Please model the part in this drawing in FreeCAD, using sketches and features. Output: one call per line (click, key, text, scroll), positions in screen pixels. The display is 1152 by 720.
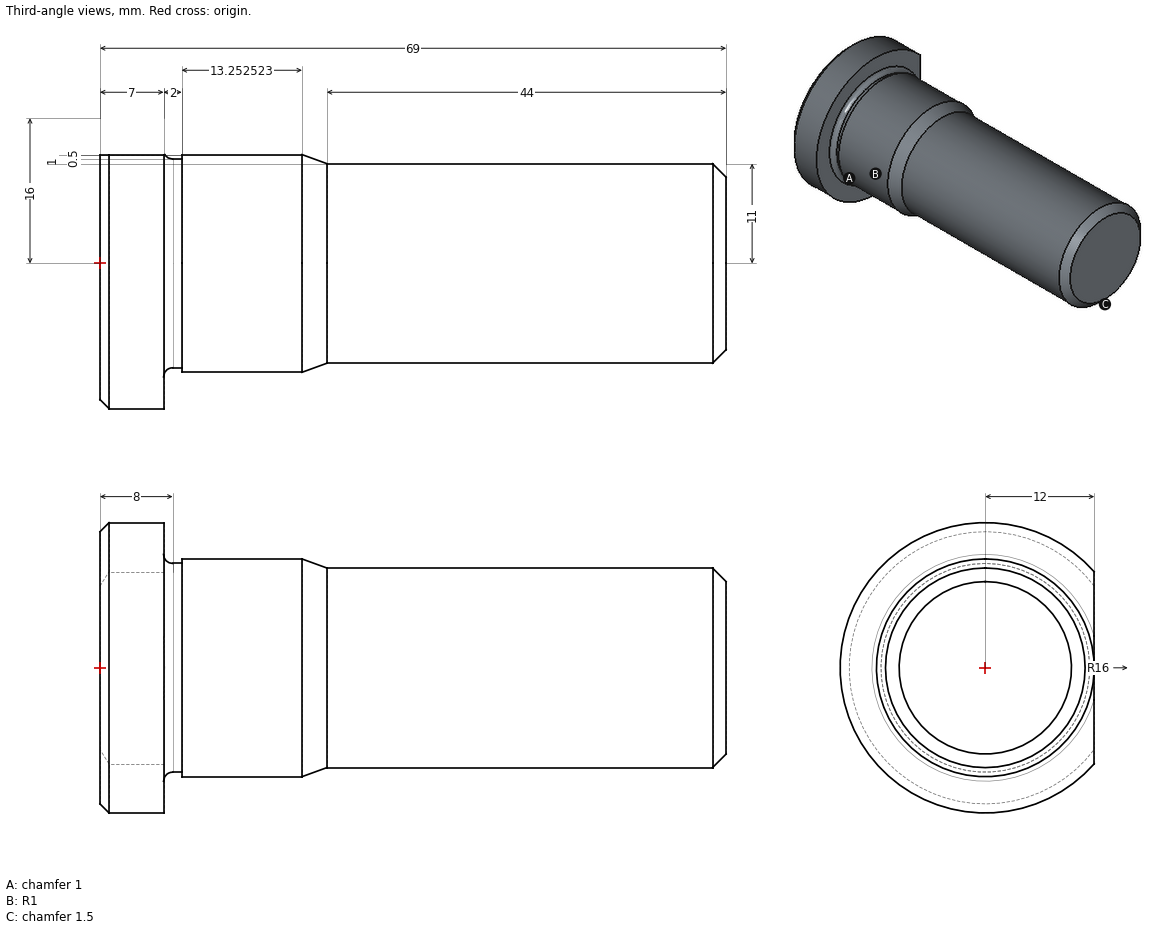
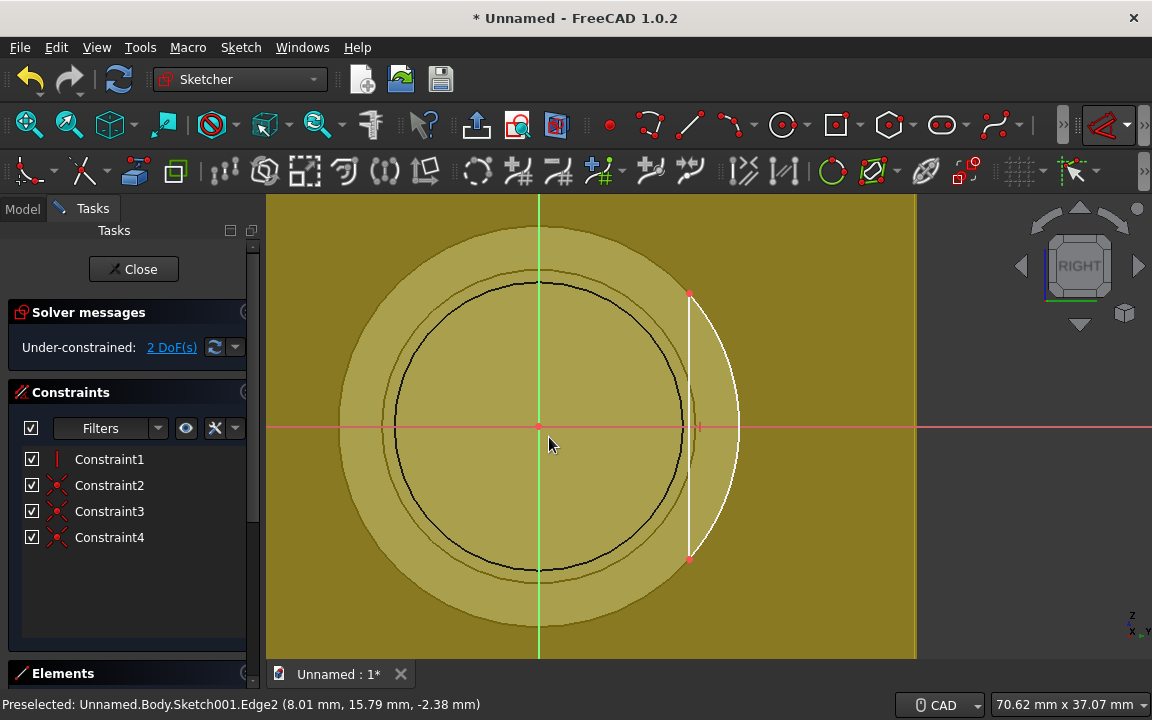
click(1102, 126)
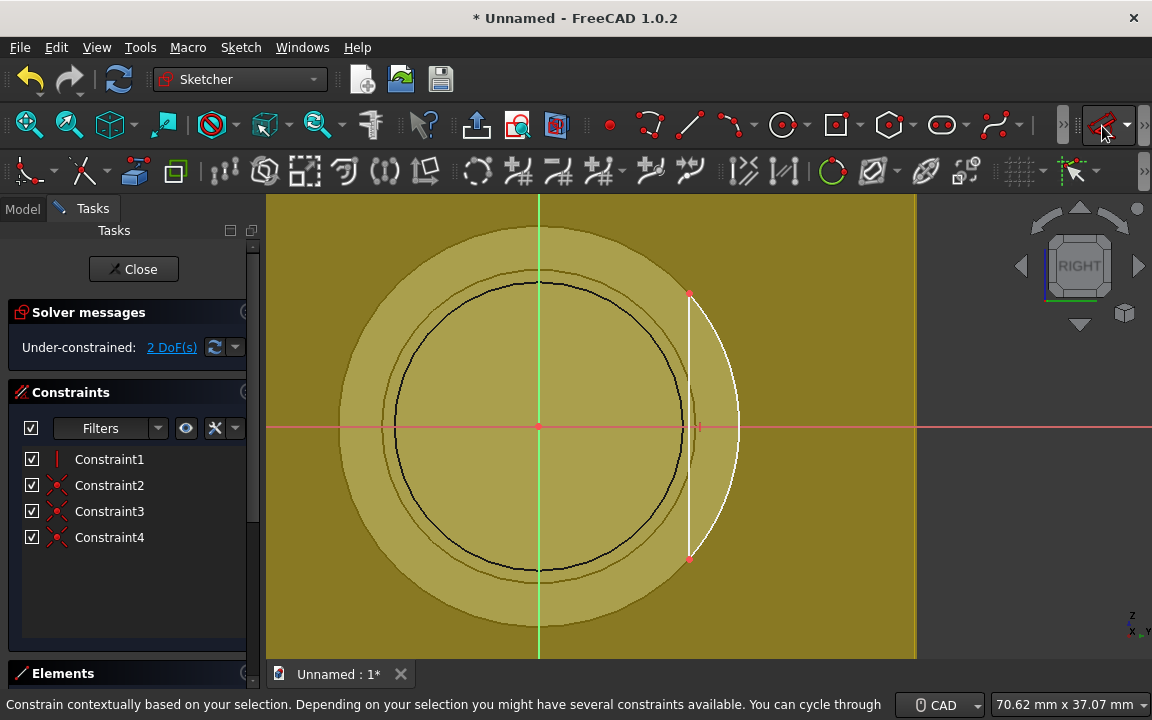
click(731, 484)
click(762, 493)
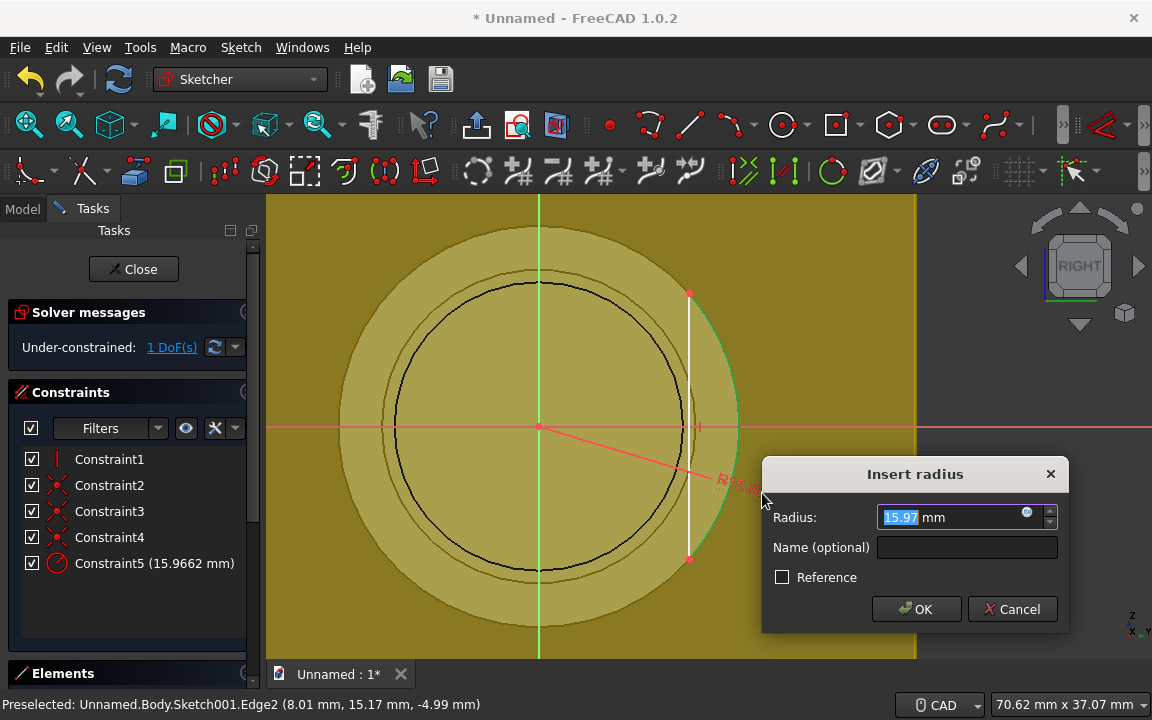
text(16)
key(Return)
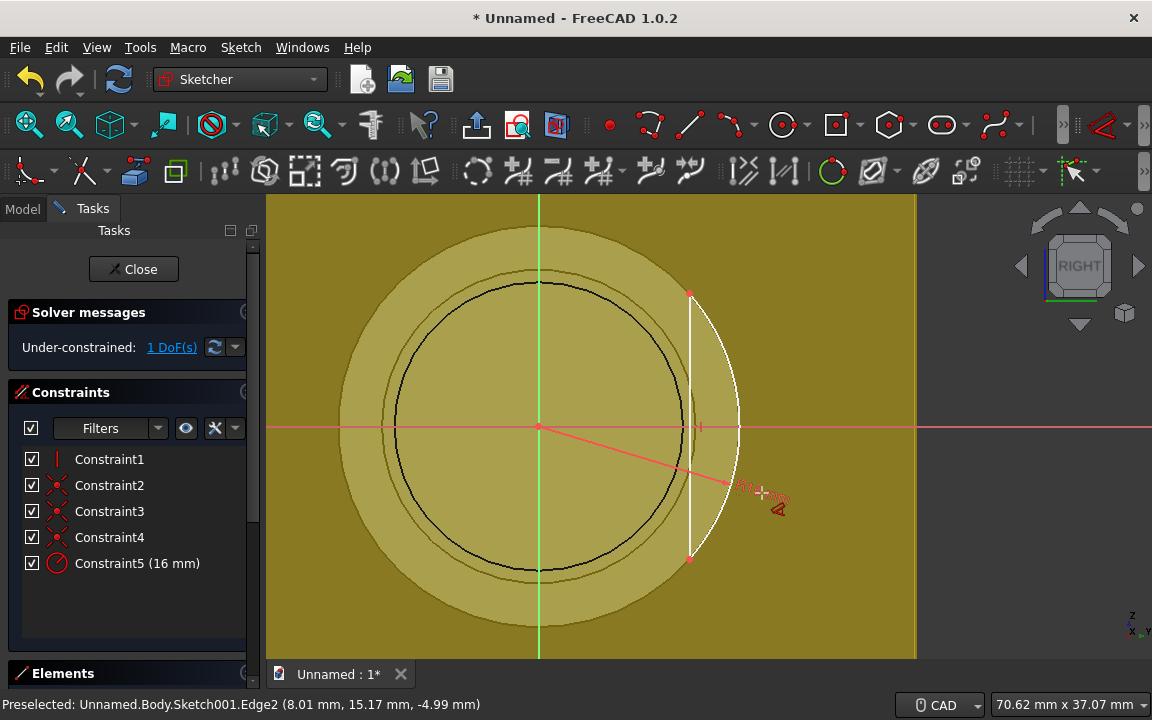
click(690, 294)
click(614, 260)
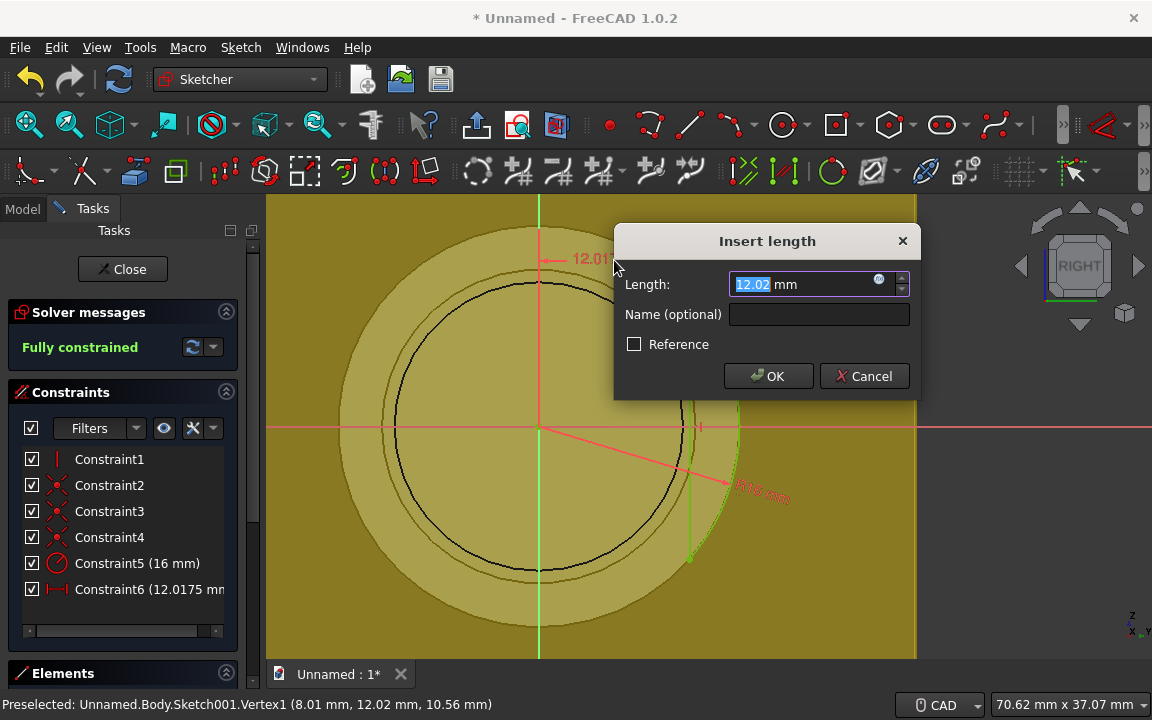
text(12)
key(Return)
key(Escape)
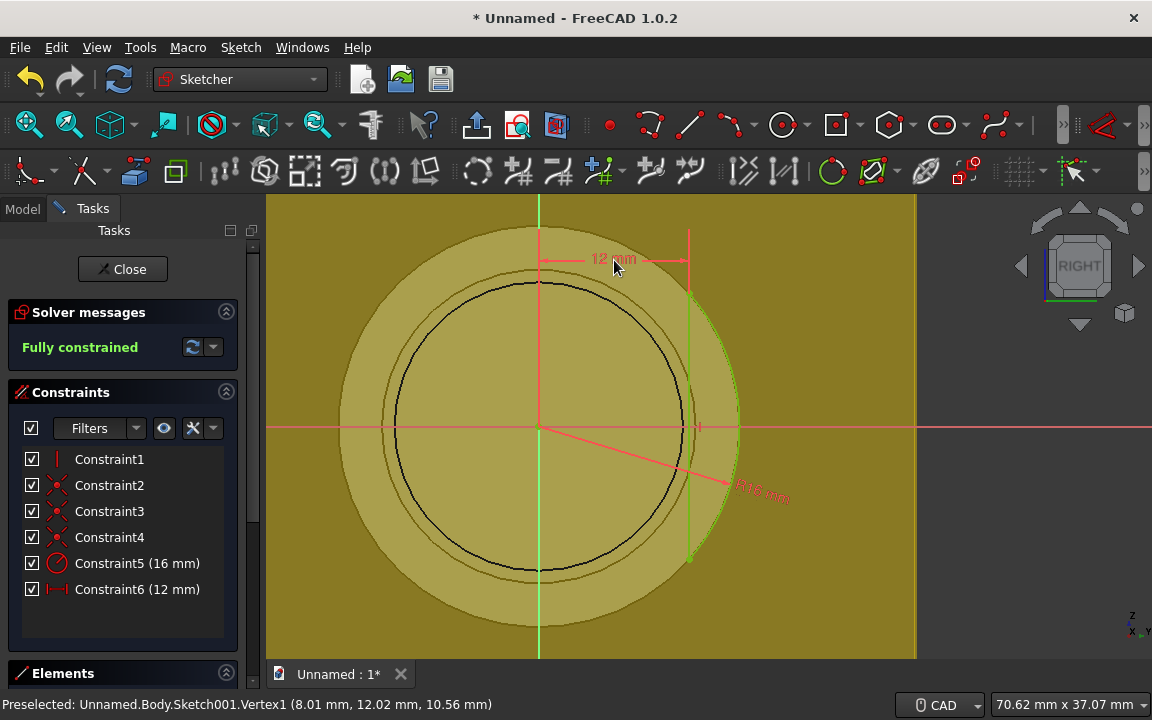
click(123, 269)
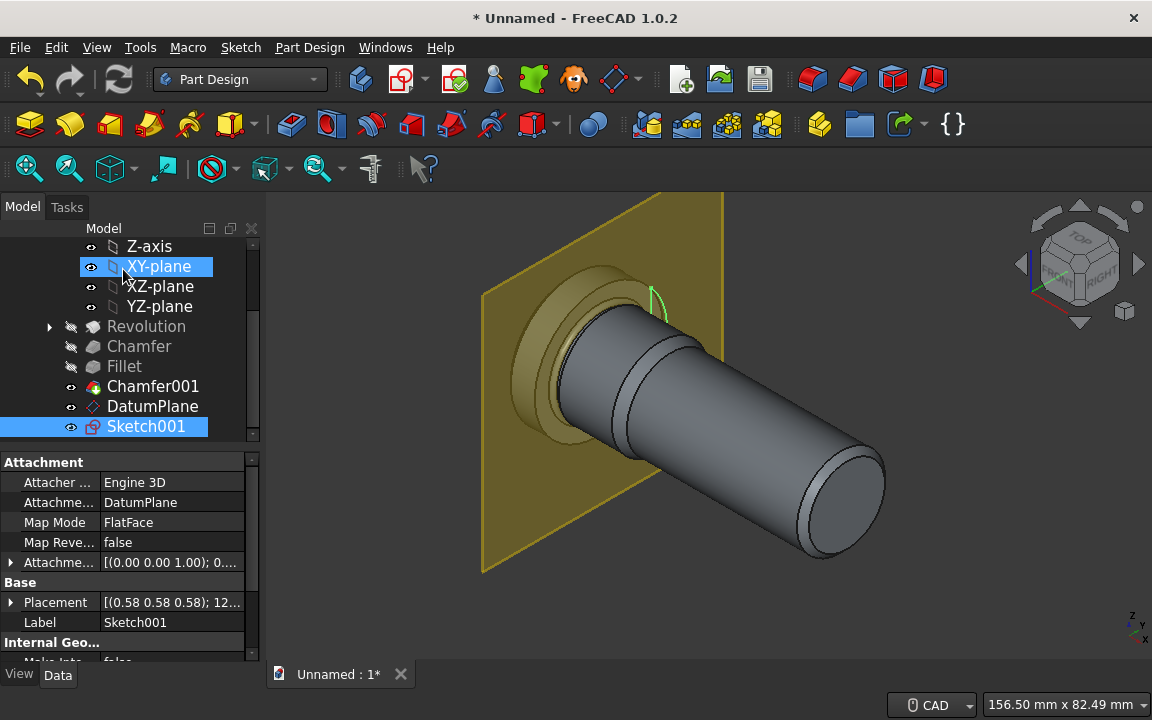
click(292, 124)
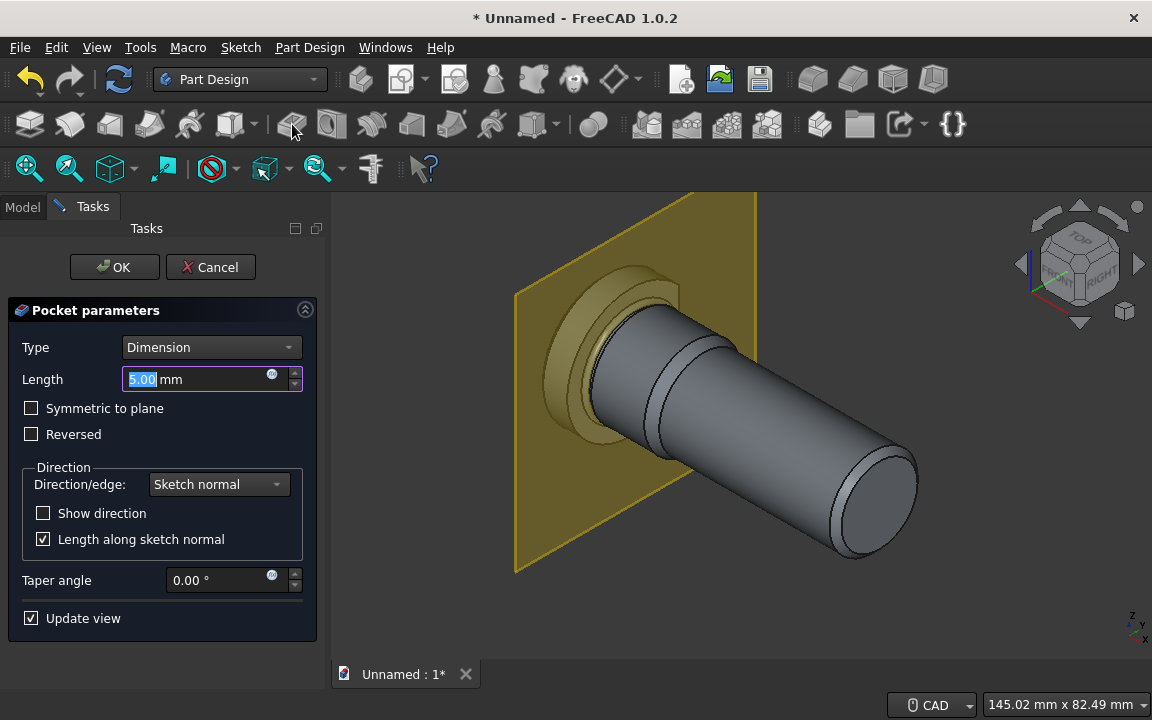
text(8)
key(Tab)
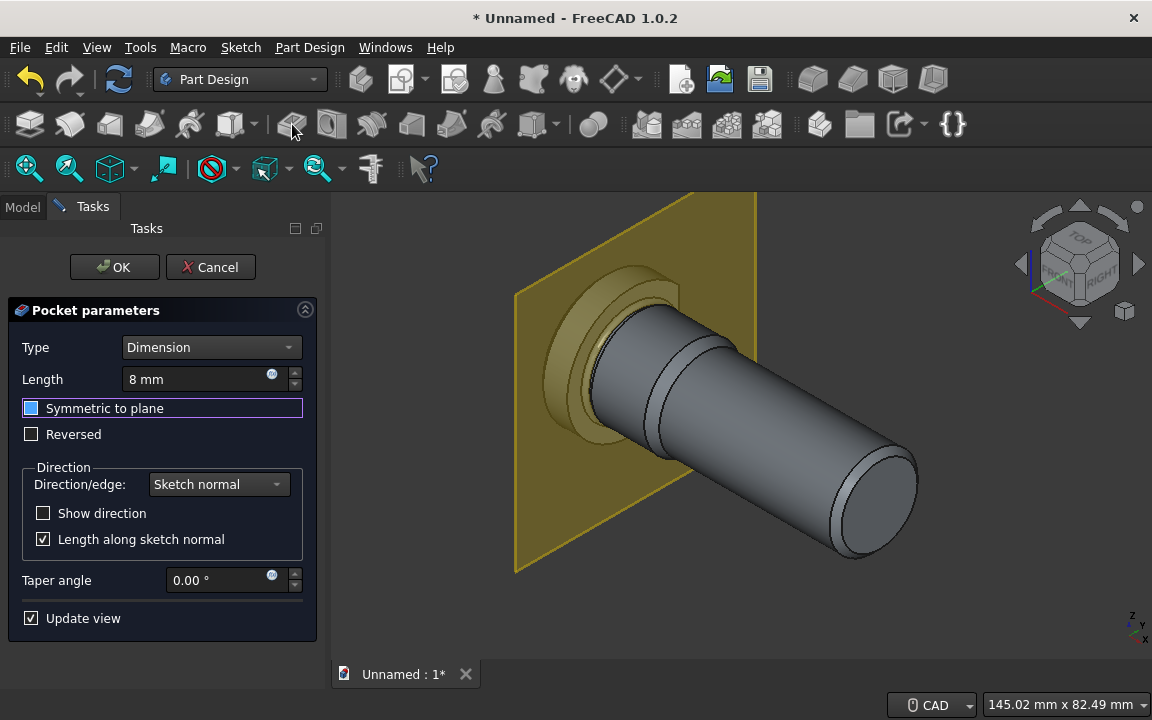
click(115, 267)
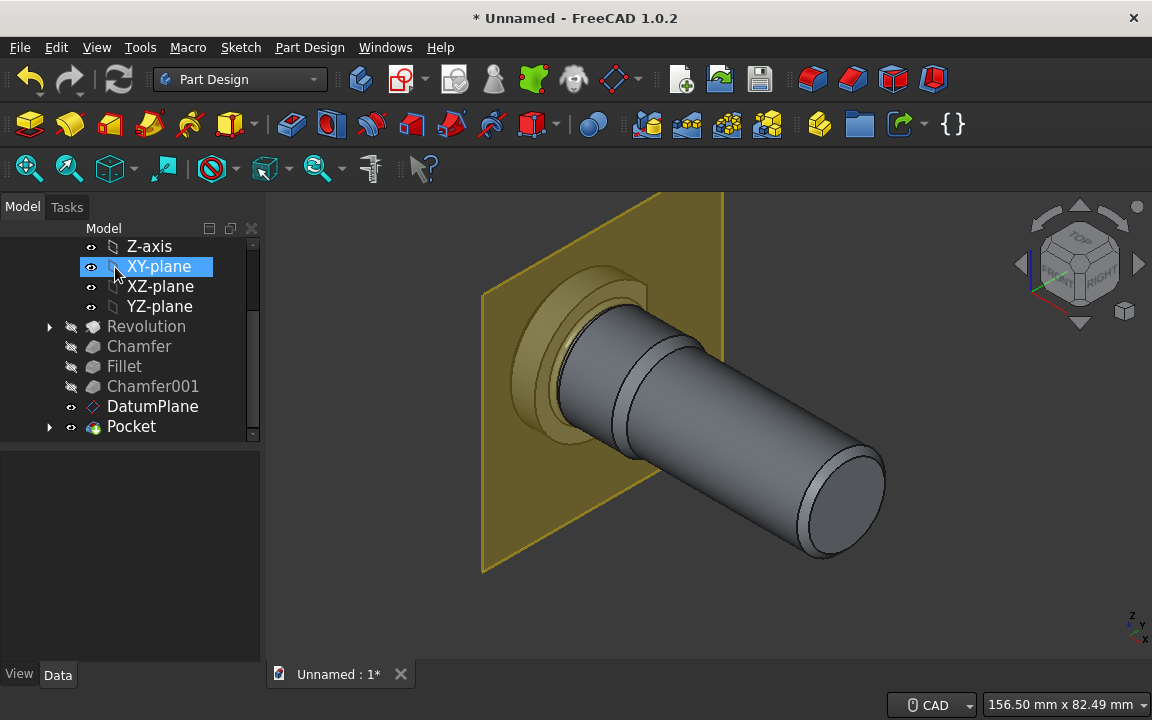
click(116, 407)
key(space)